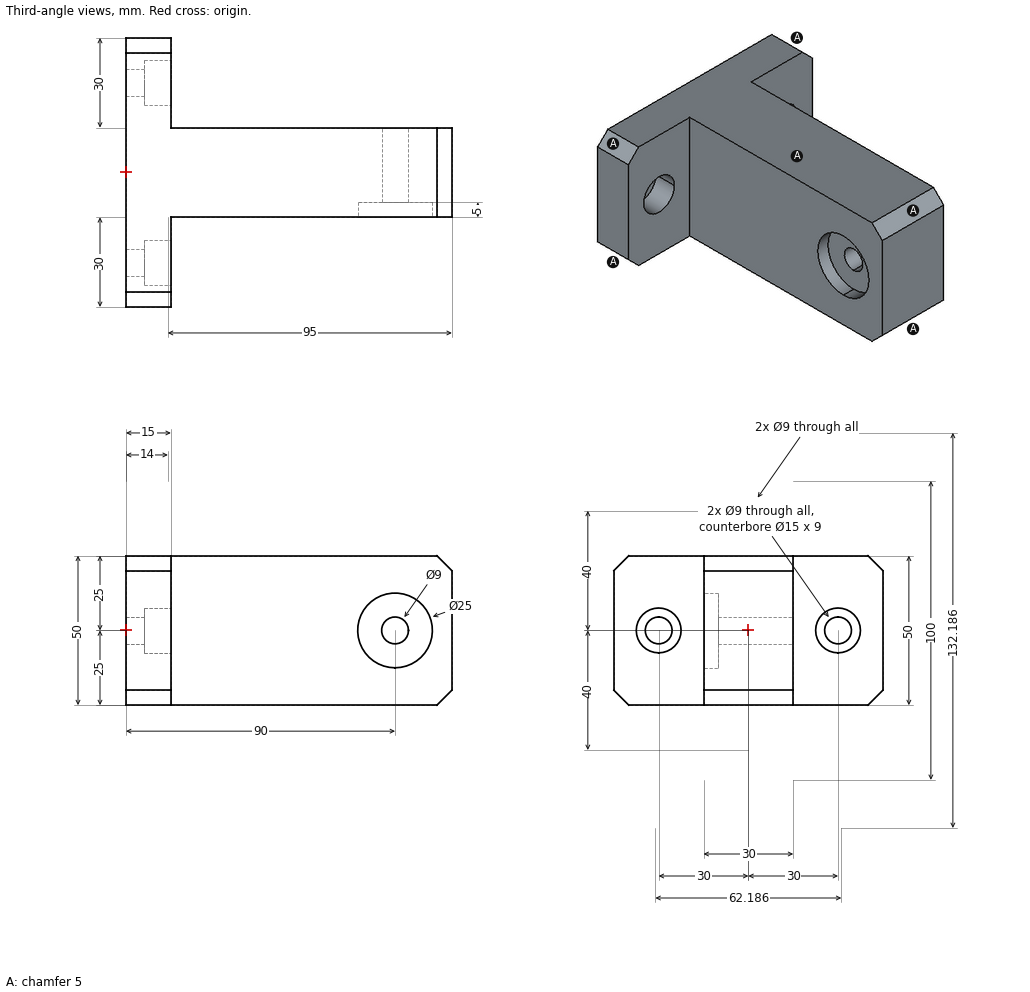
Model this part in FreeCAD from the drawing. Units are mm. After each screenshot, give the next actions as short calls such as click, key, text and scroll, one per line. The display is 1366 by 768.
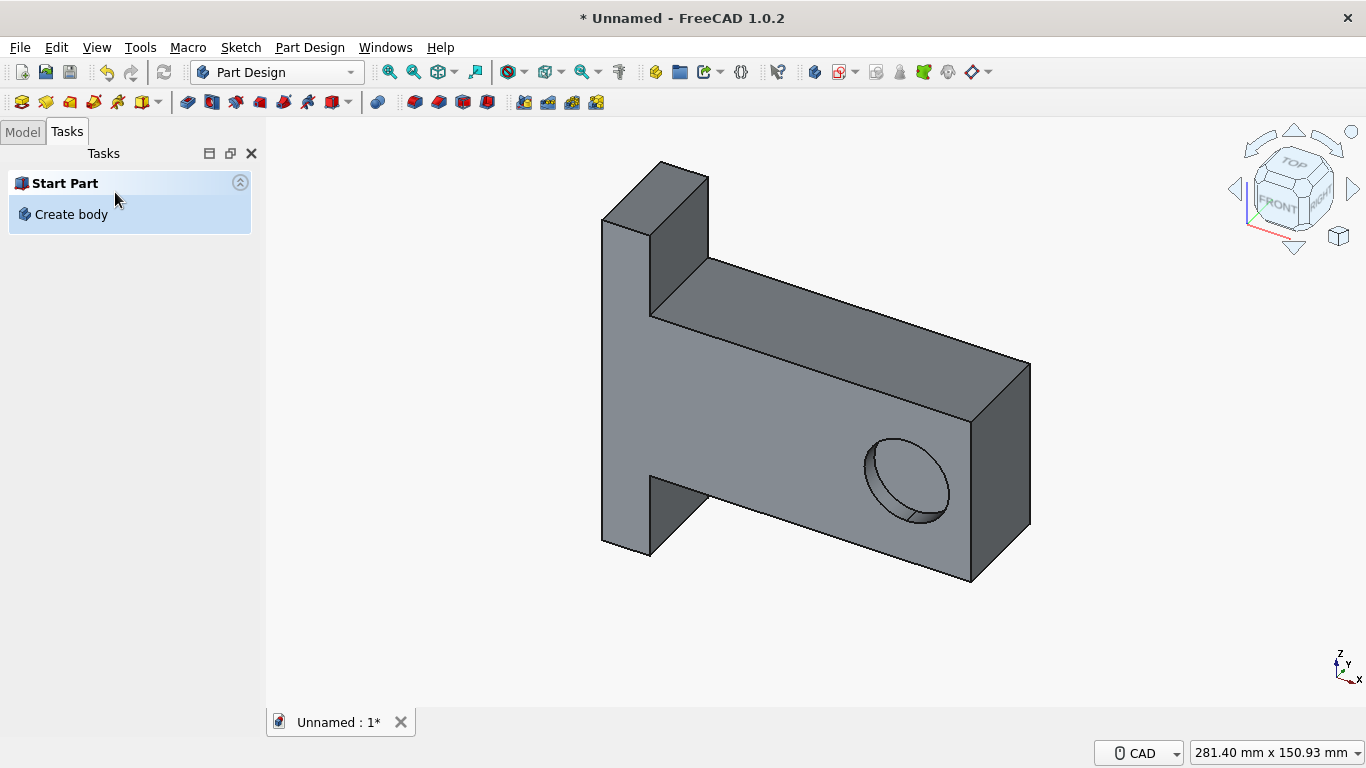
click(734, 423)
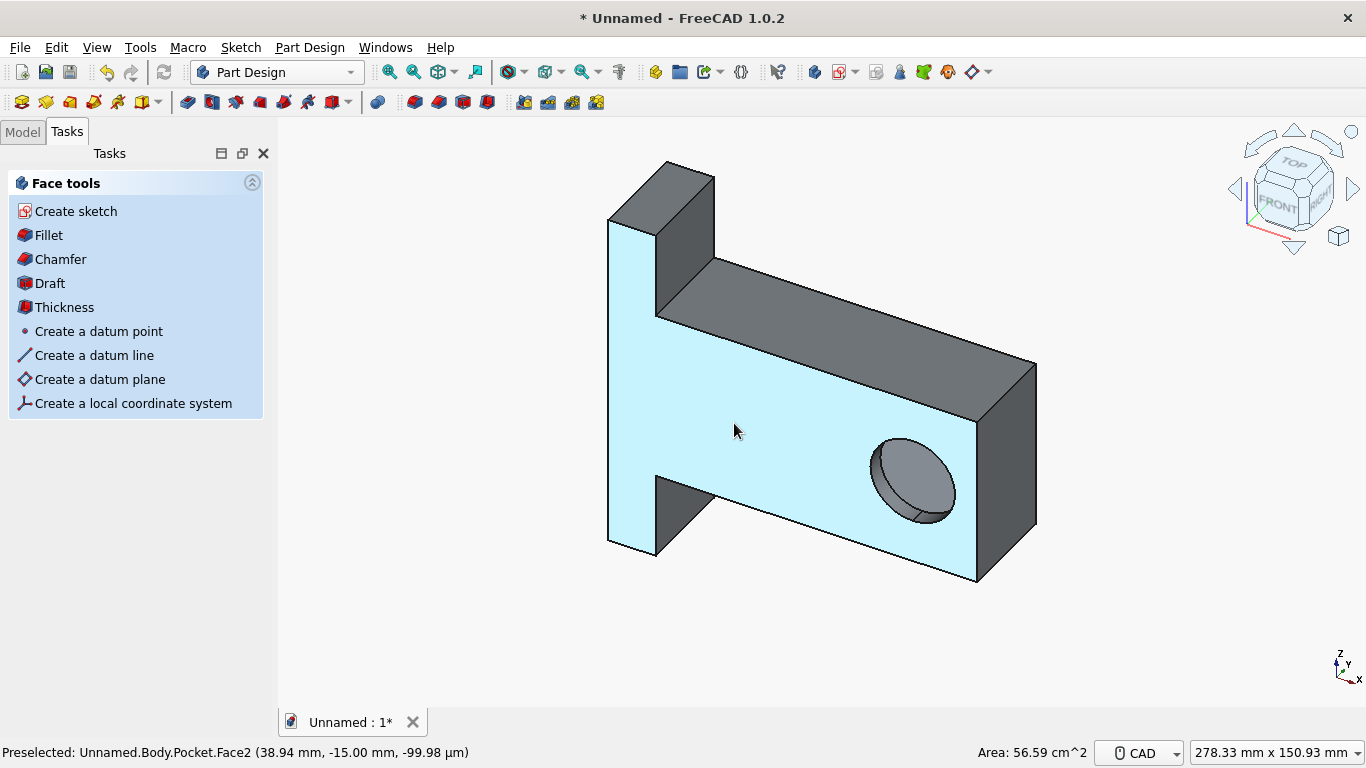
click(840, 72)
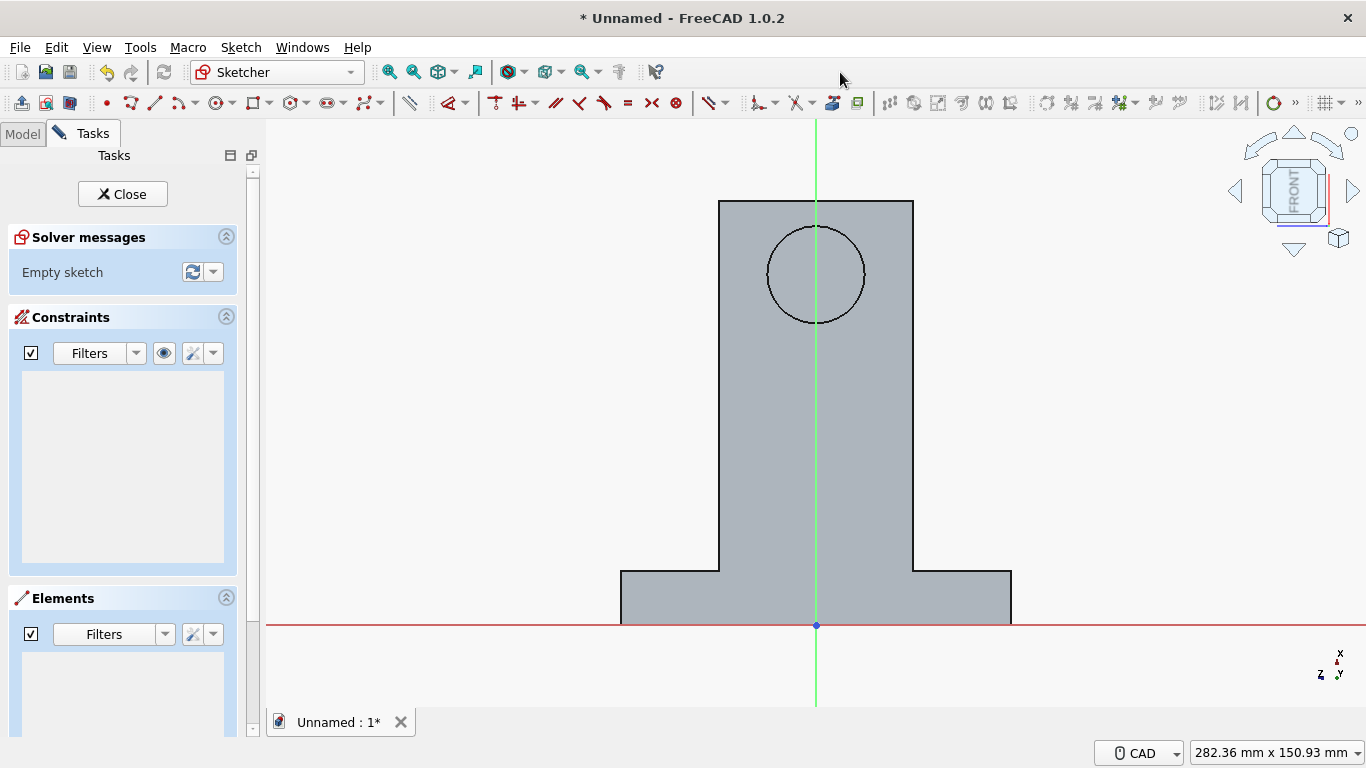
scroll(823, 261, up, 12)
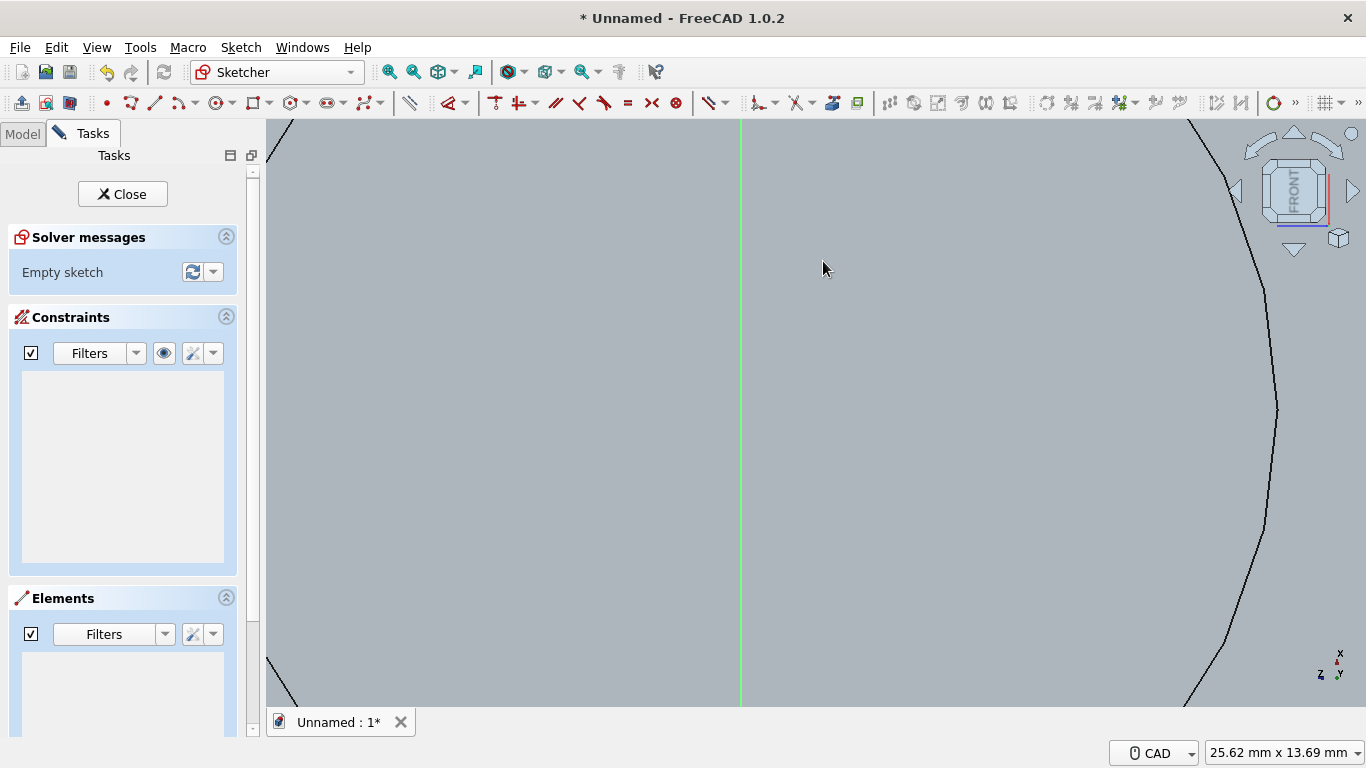
key(g)
key(c)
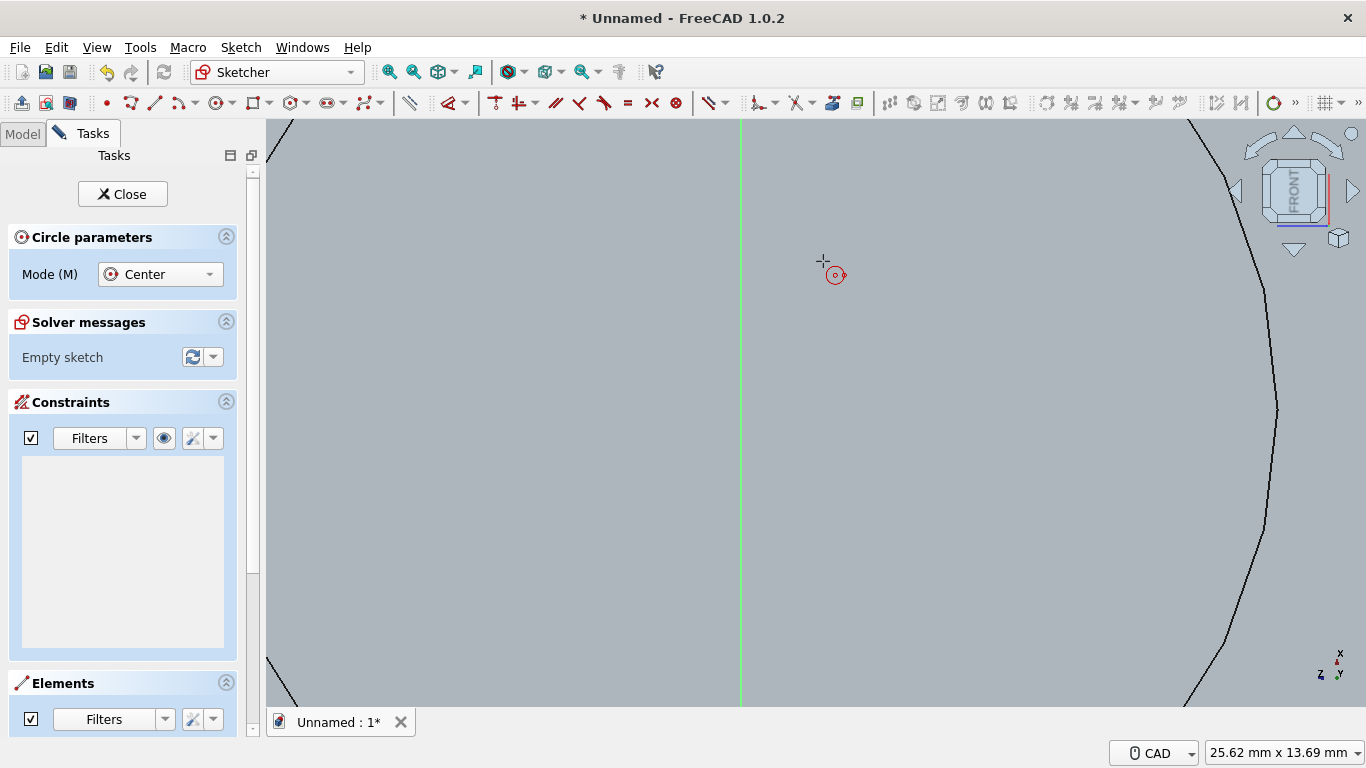
click(741, 410)
move(877, 273)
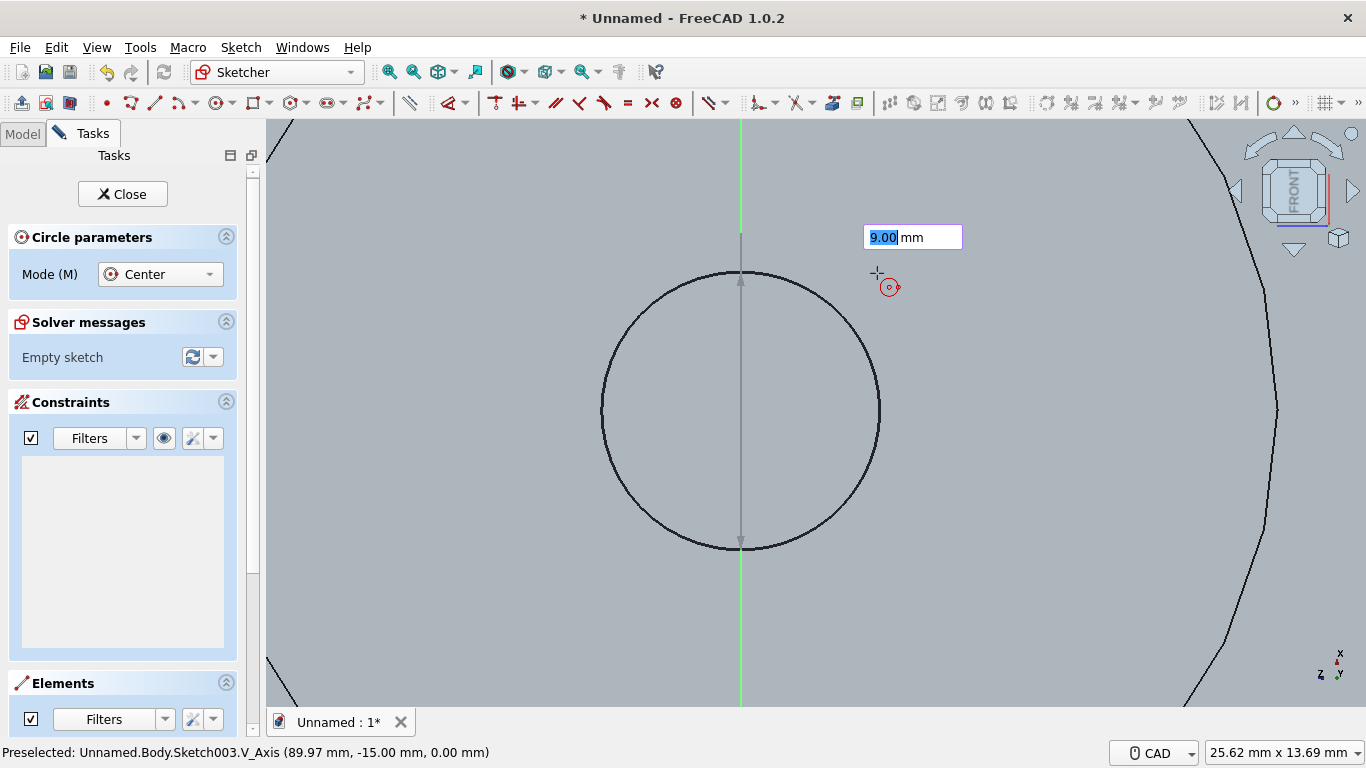
text(9)
key(Return)
key(Escape)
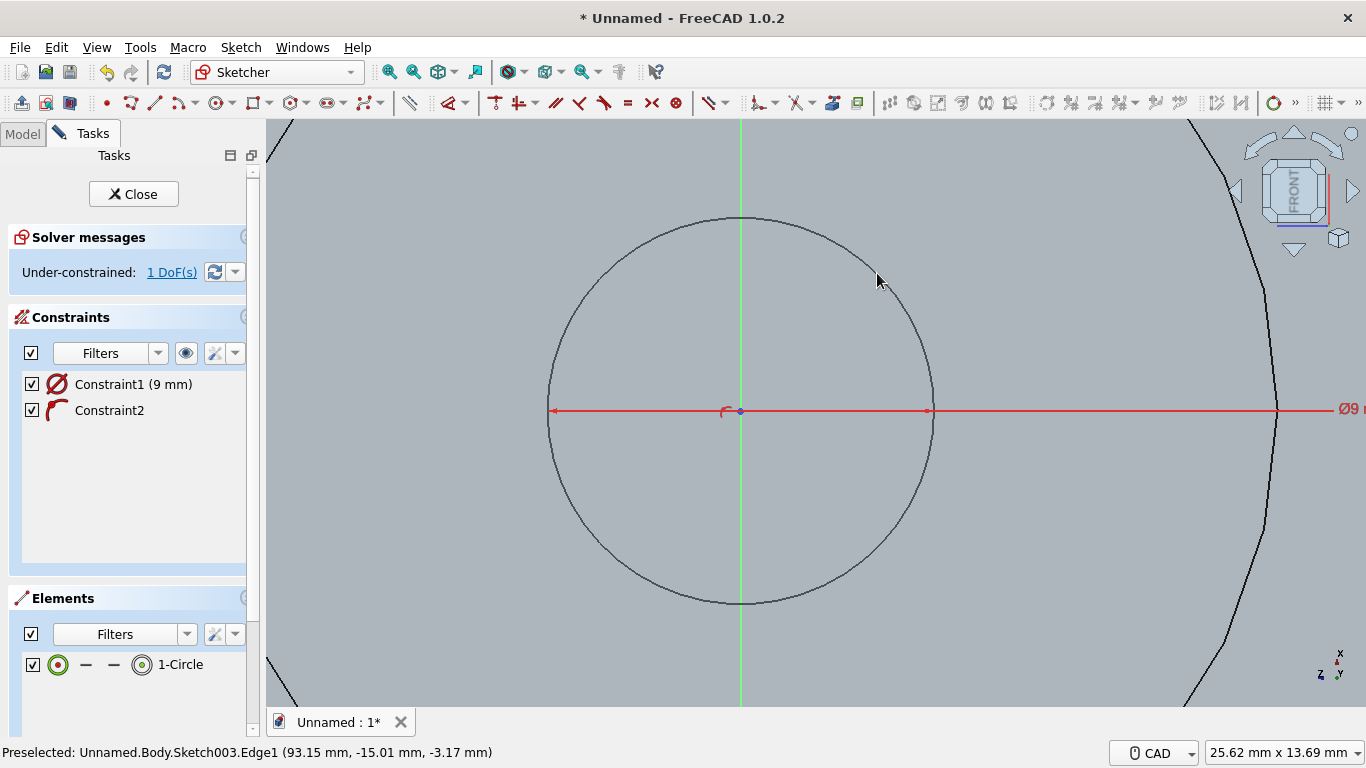
click(448, 104)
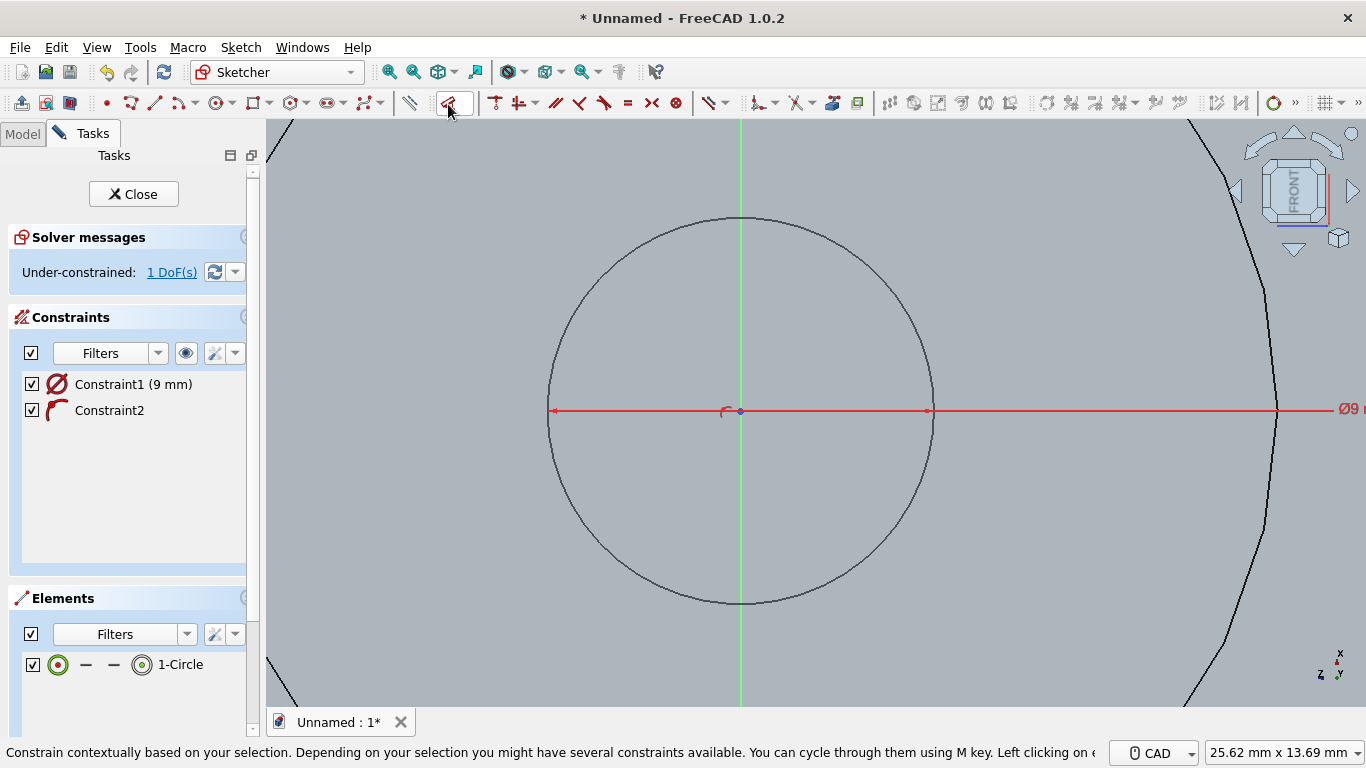
click(741, 411)
click(775, 545)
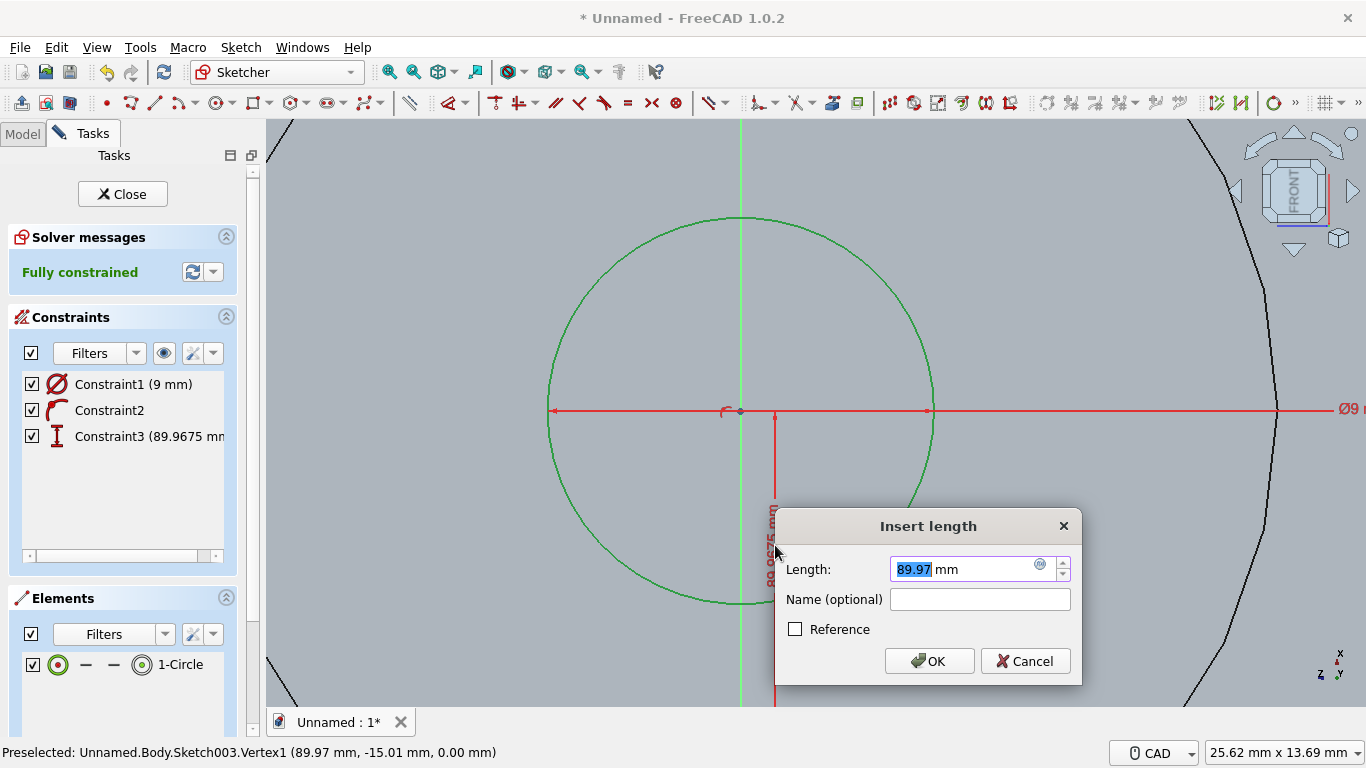
text(90)
key(Return)
key(Escape)